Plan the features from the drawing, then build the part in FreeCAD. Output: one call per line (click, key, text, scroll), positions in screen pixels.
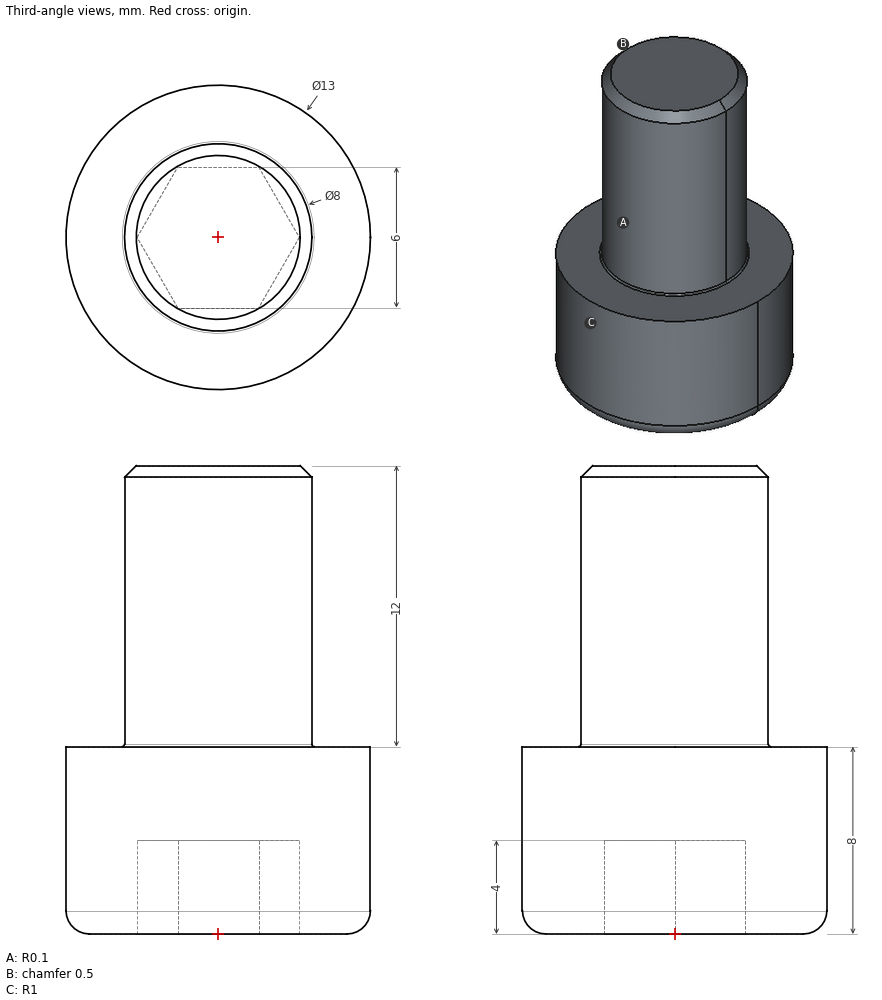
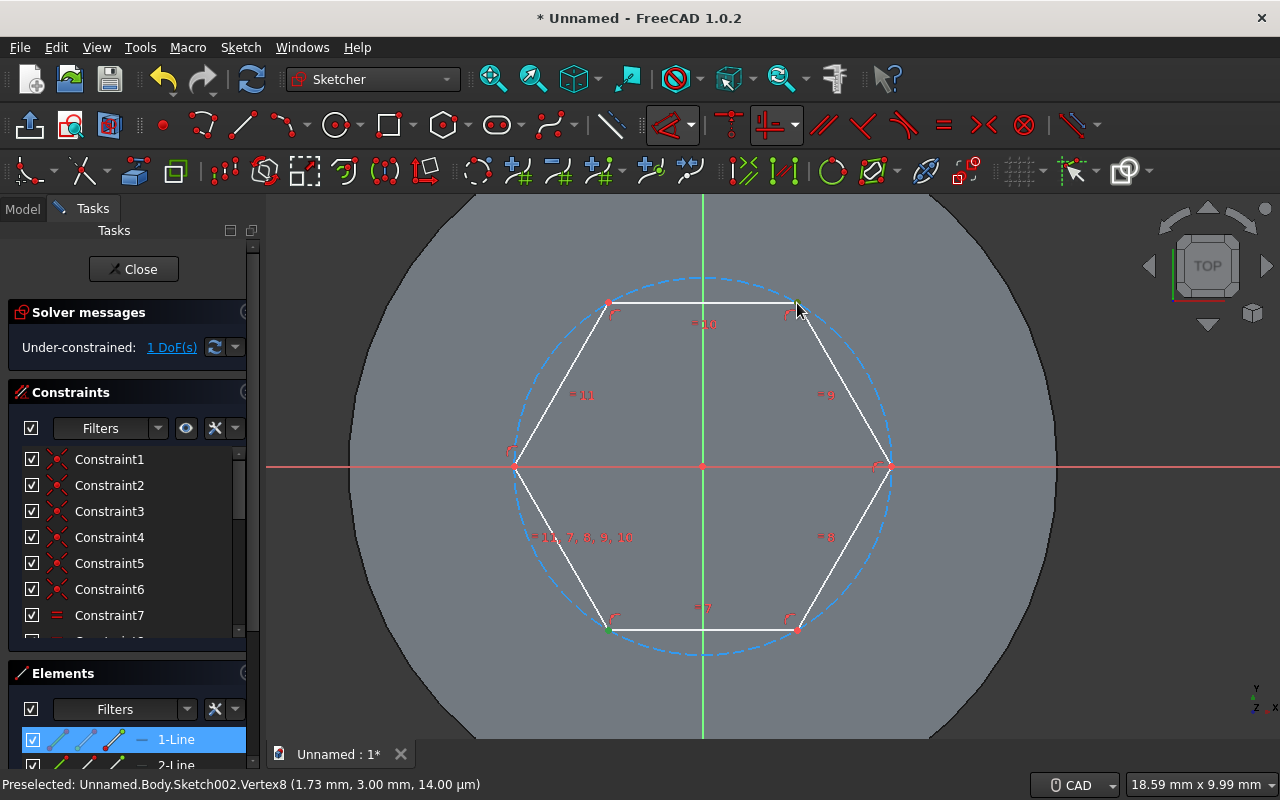
key(i)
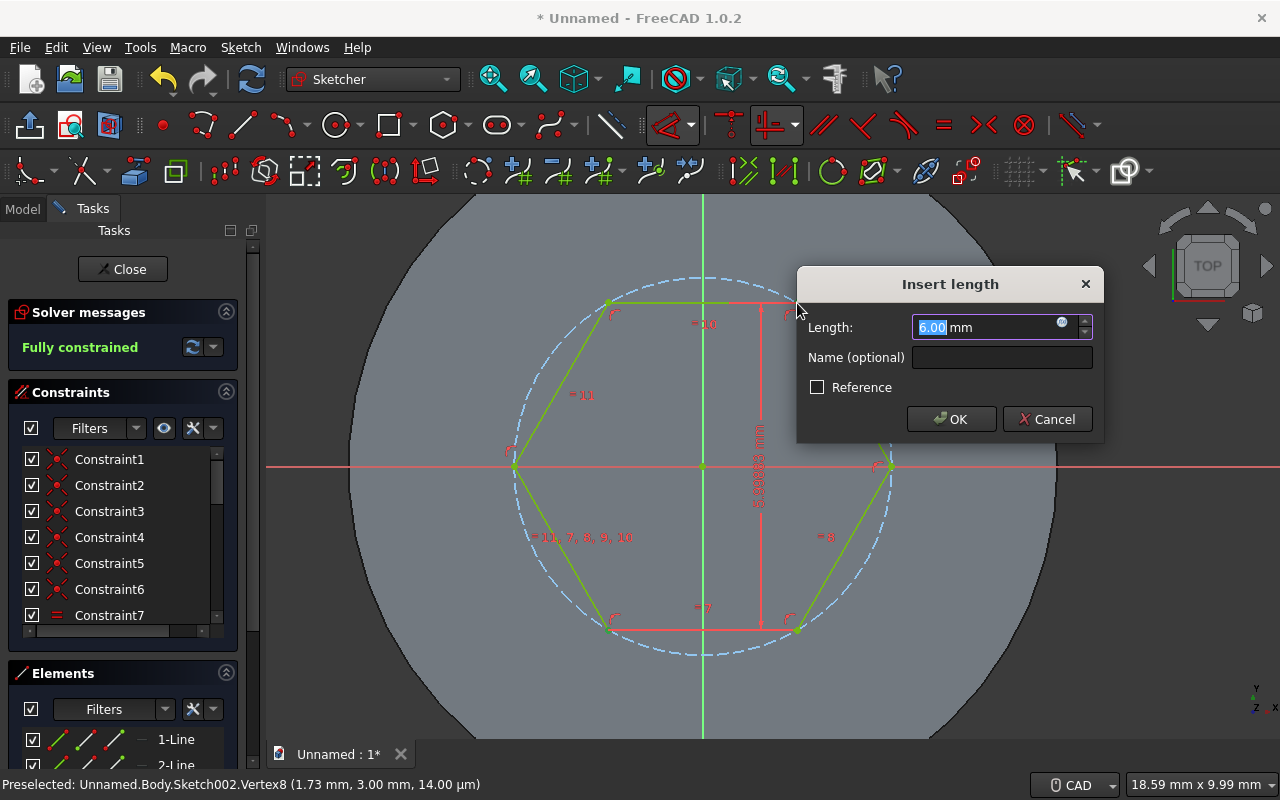
text(6)
key(Return)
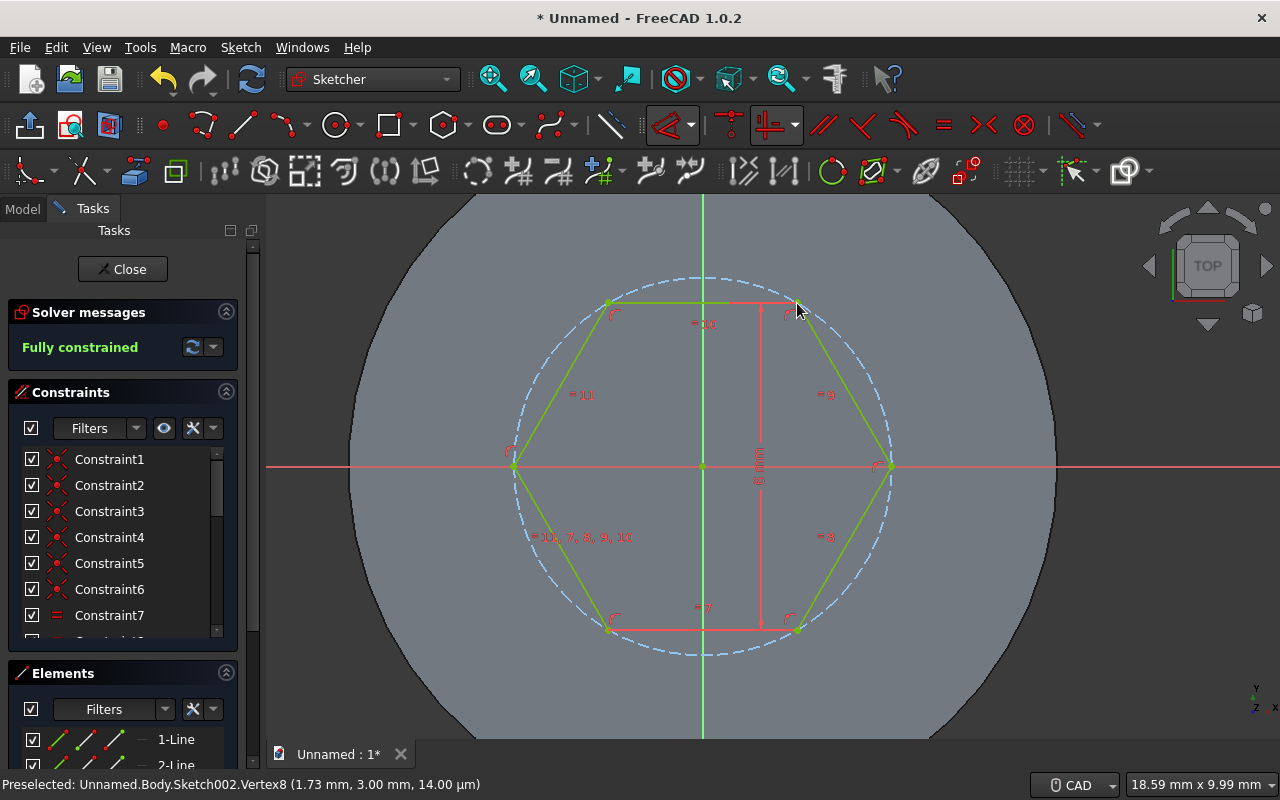
click(123, 269)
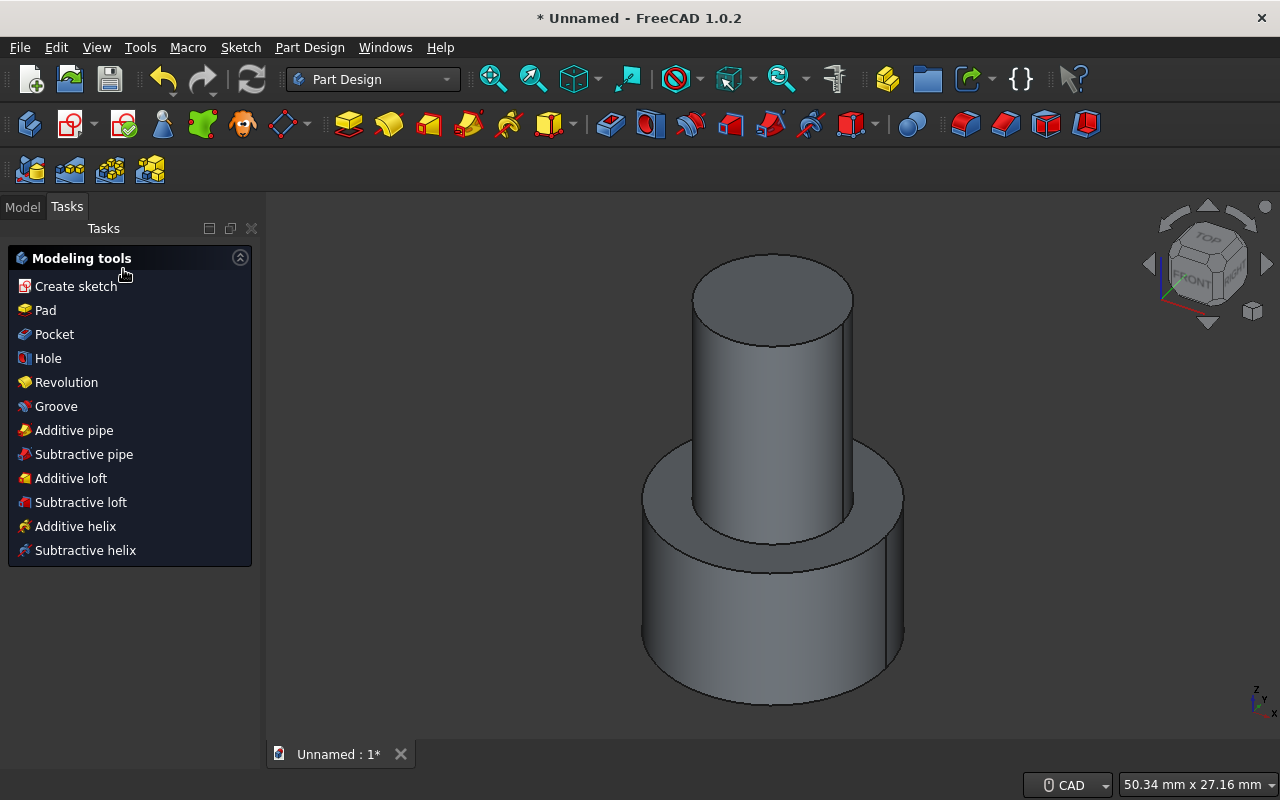
click(612, 124)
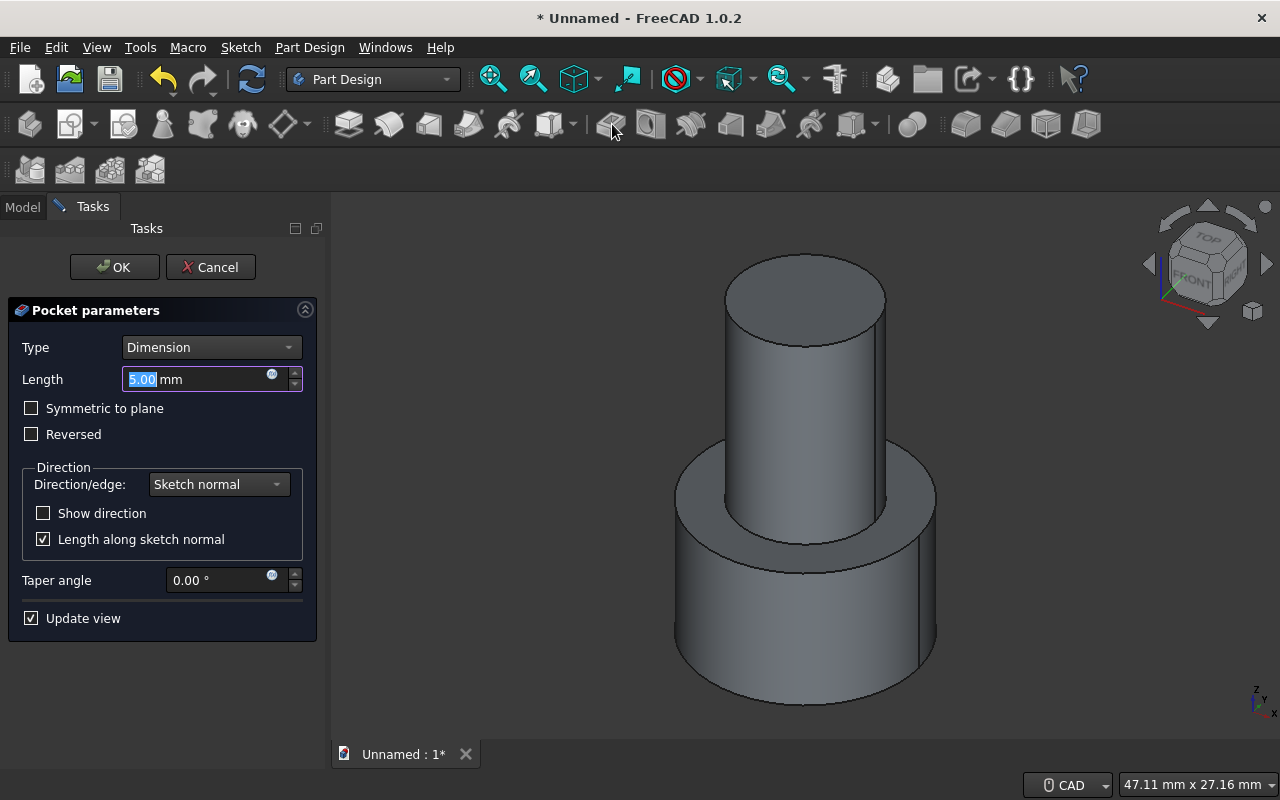
text(4)
key(Tab)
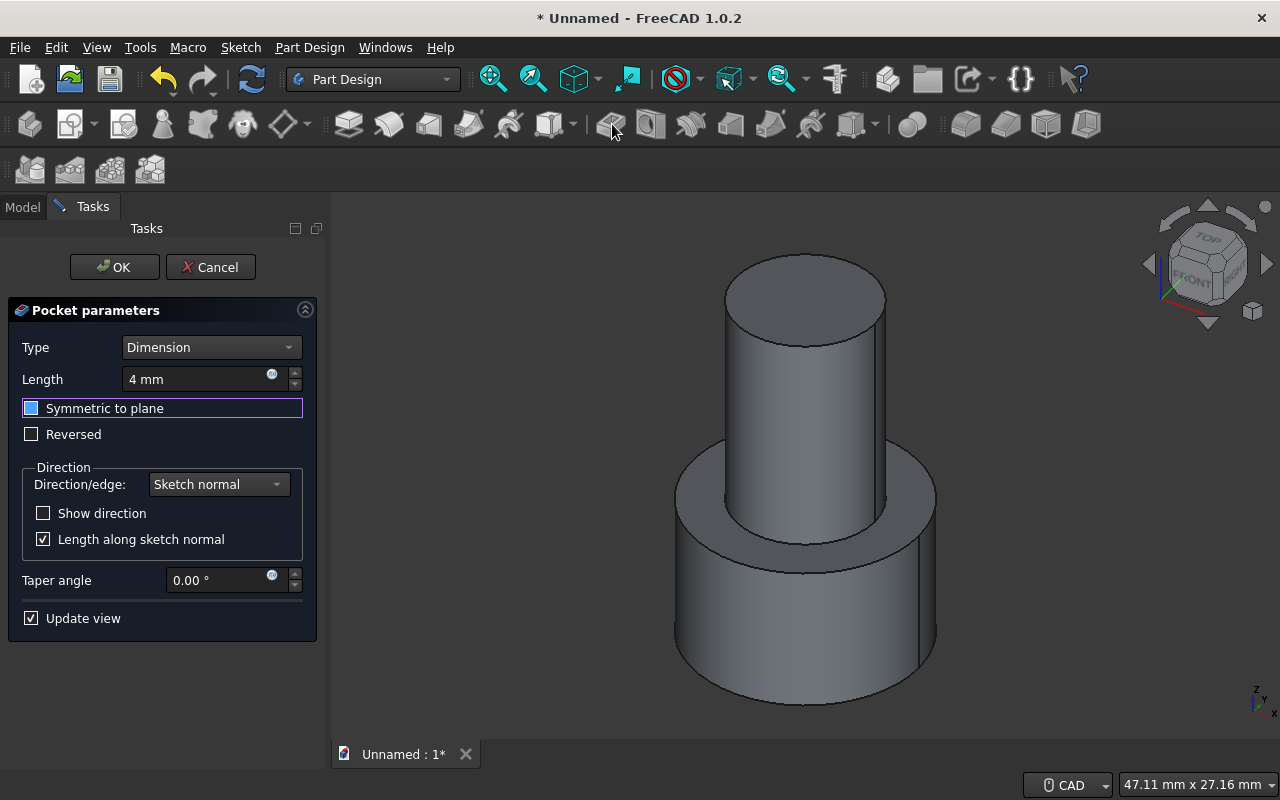
click(30, 434)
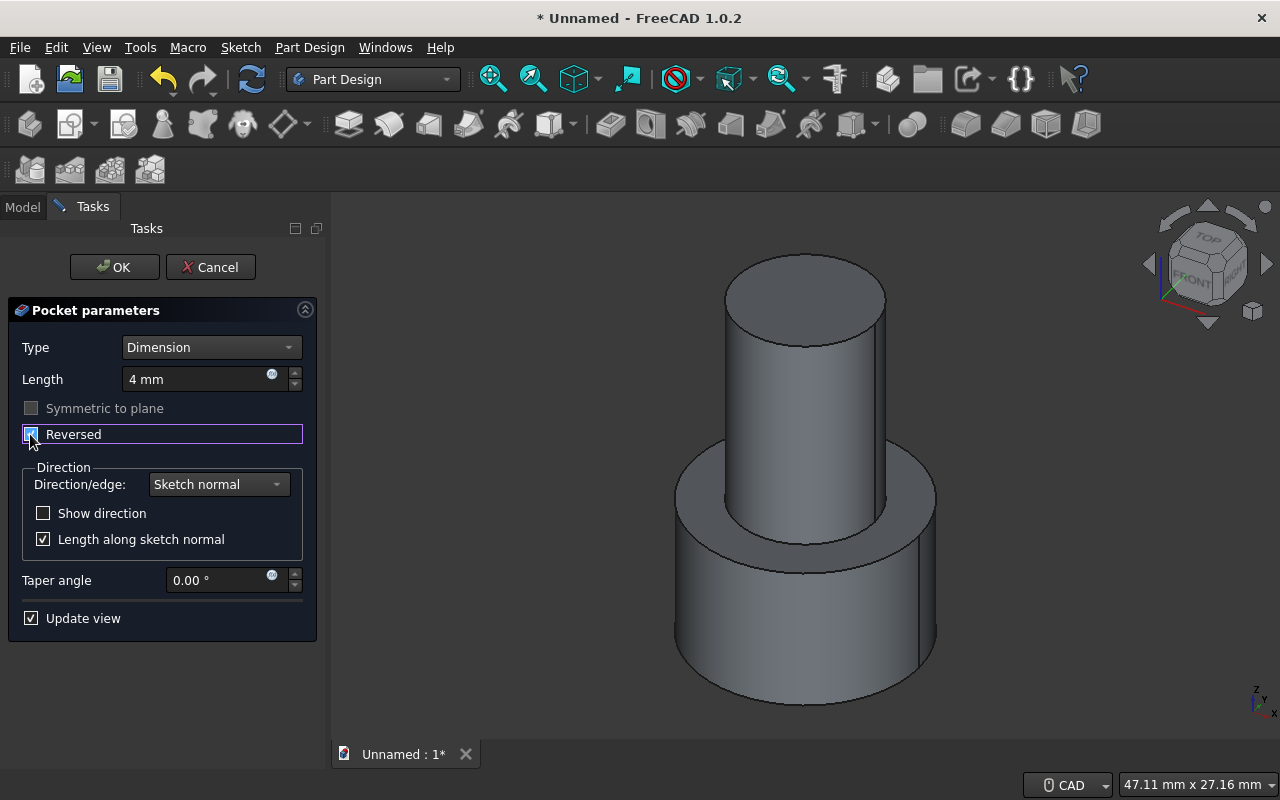
click(115, 267)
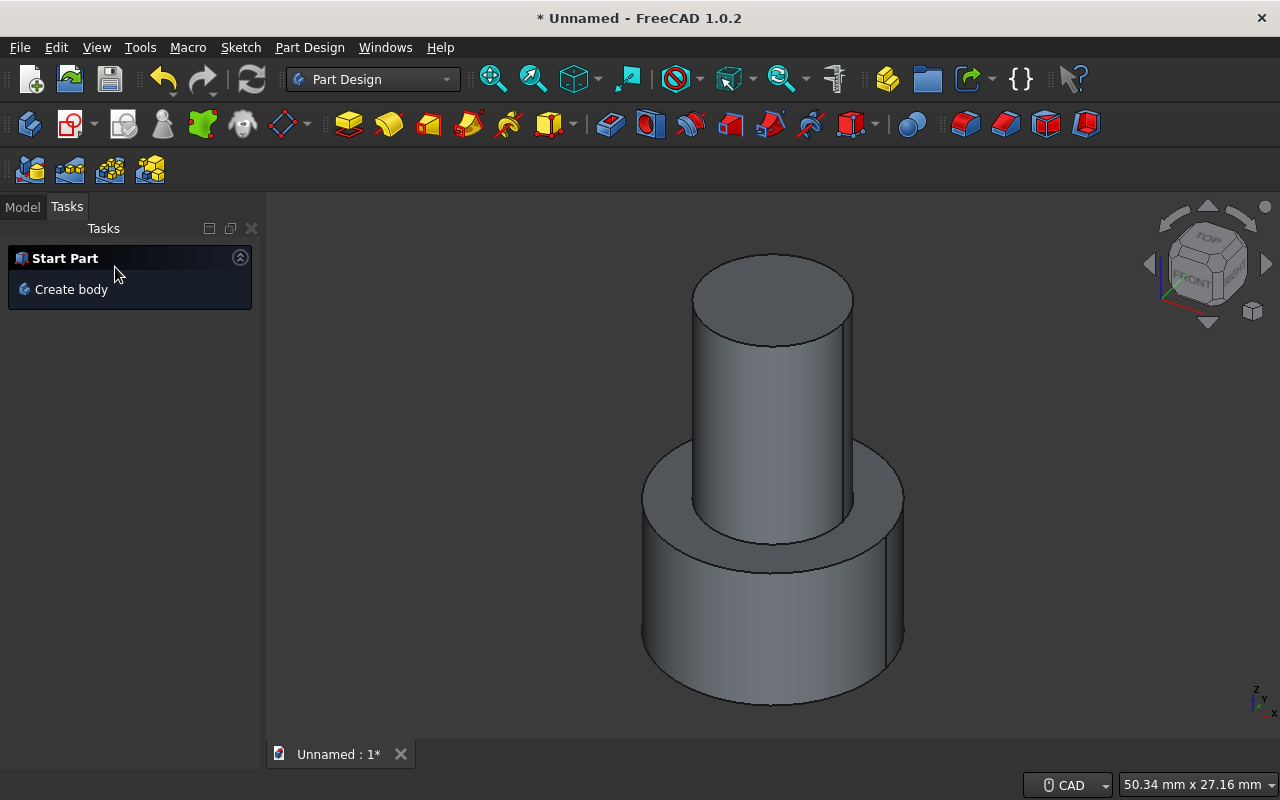
key(0)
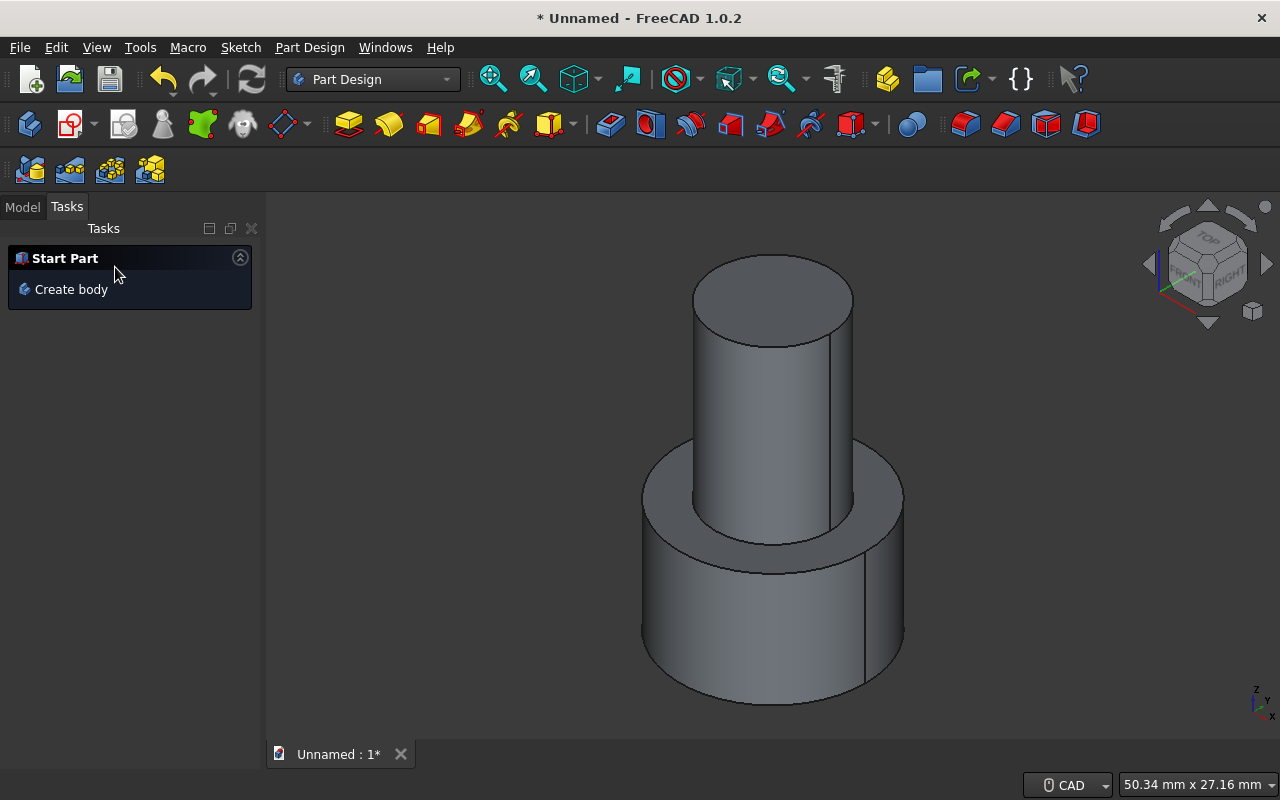
key(2)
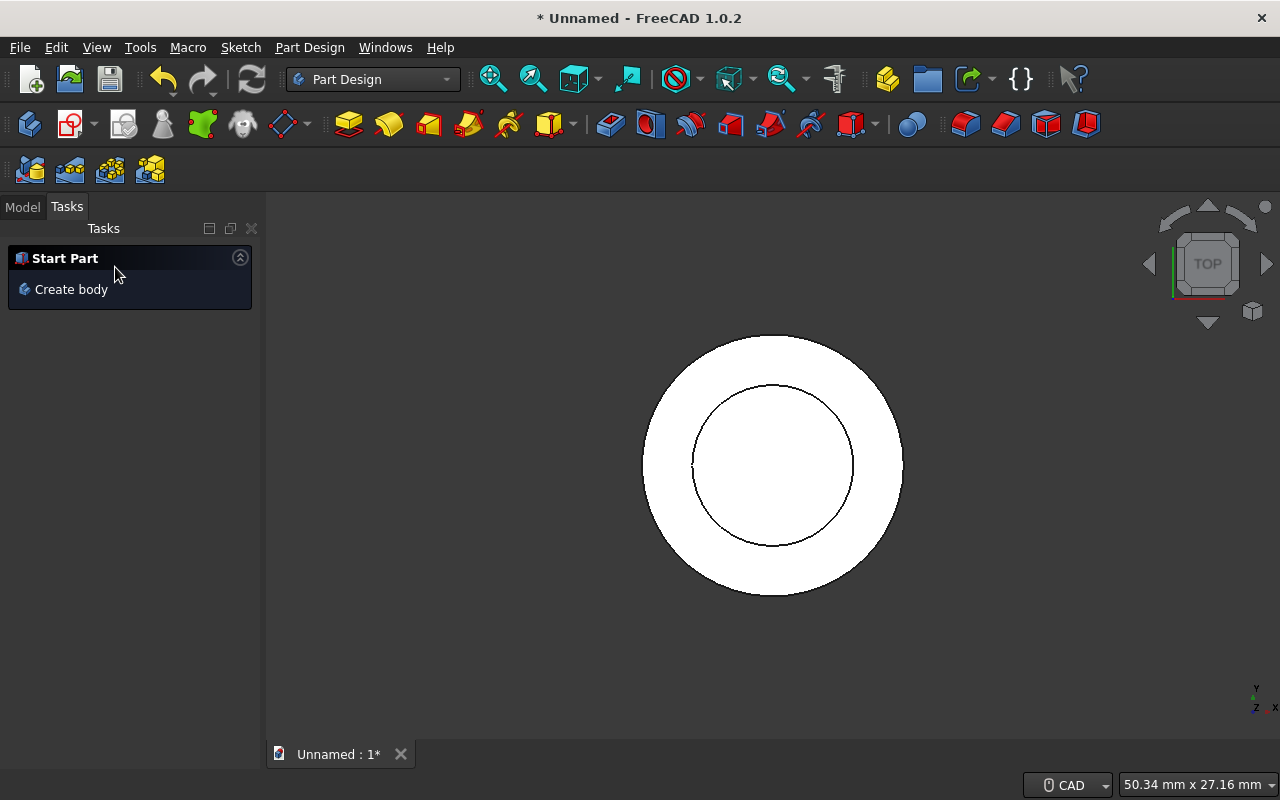
key(1)